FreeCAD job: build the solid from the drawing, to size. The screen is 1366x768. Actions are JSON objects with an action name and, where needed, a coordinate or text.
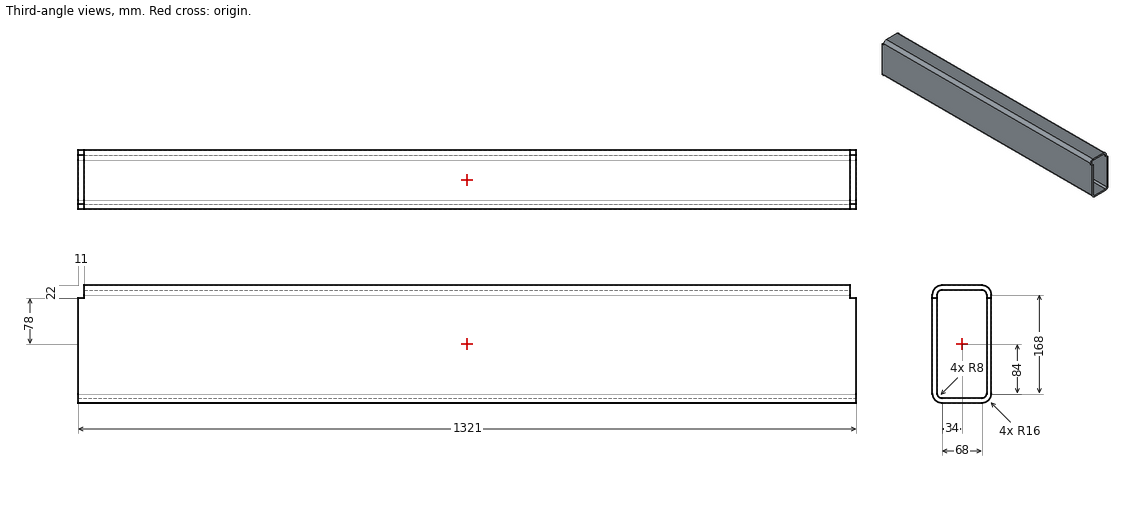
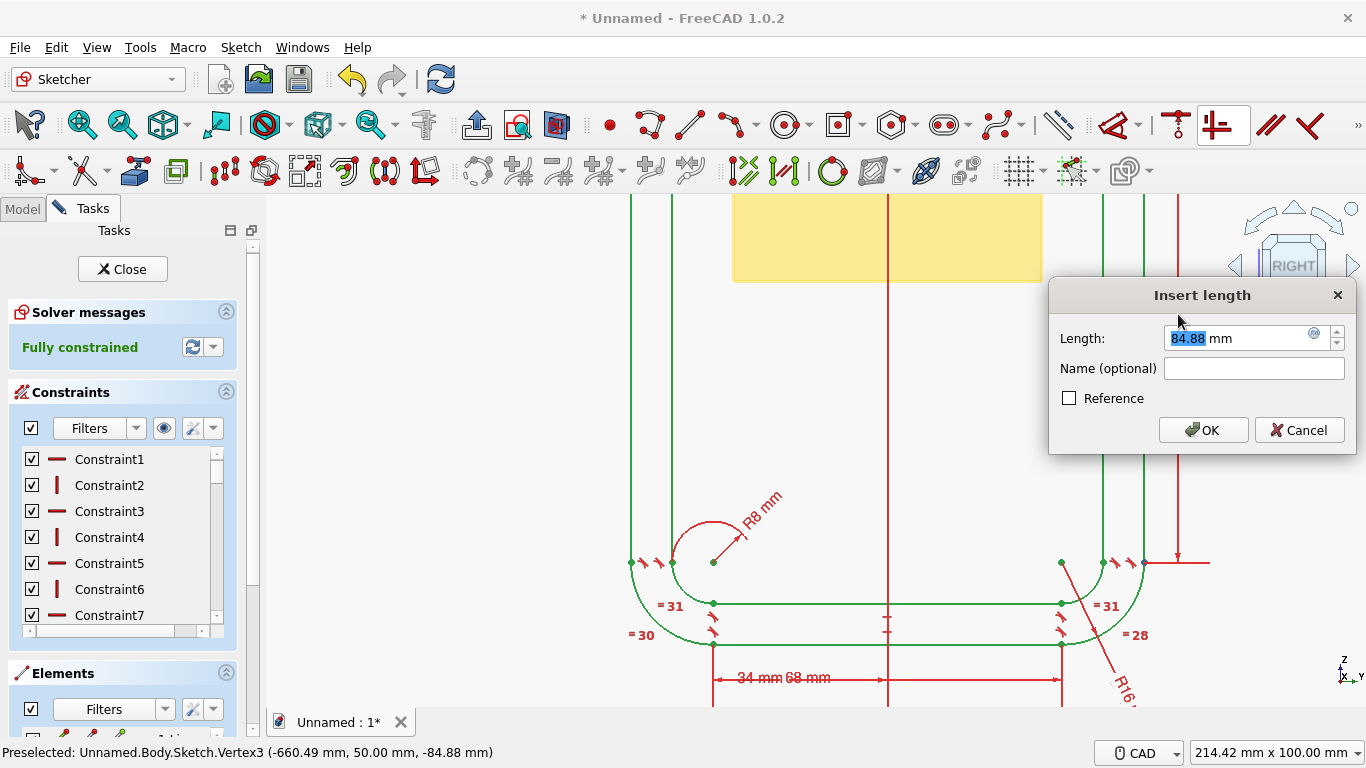
{"action": "type", "text": "84"}
{"action": "key", "text": "Return"}
{"action": "key", "text": "Escape"}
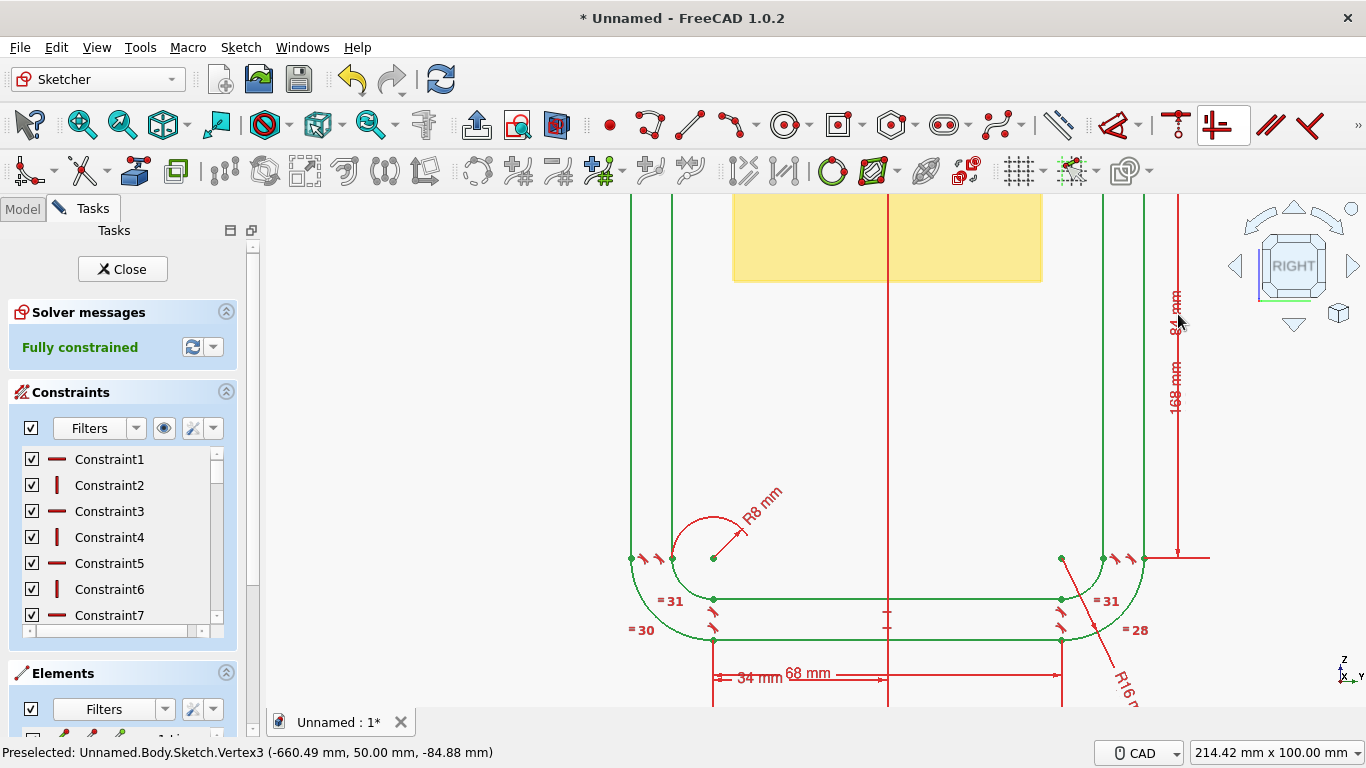
{"action": "left_click", "coordinate": [123, 269]}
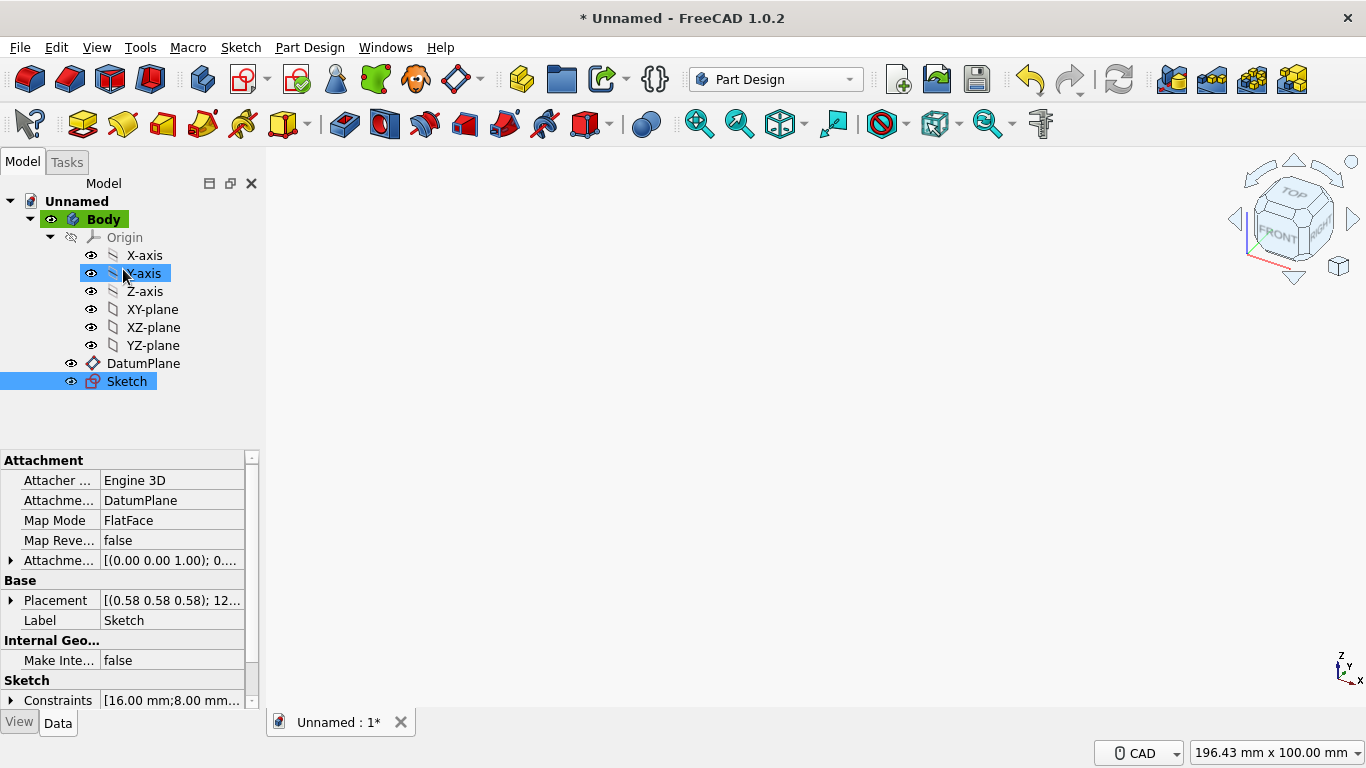
{"action": "left_click", "coordinate": [84, 124]}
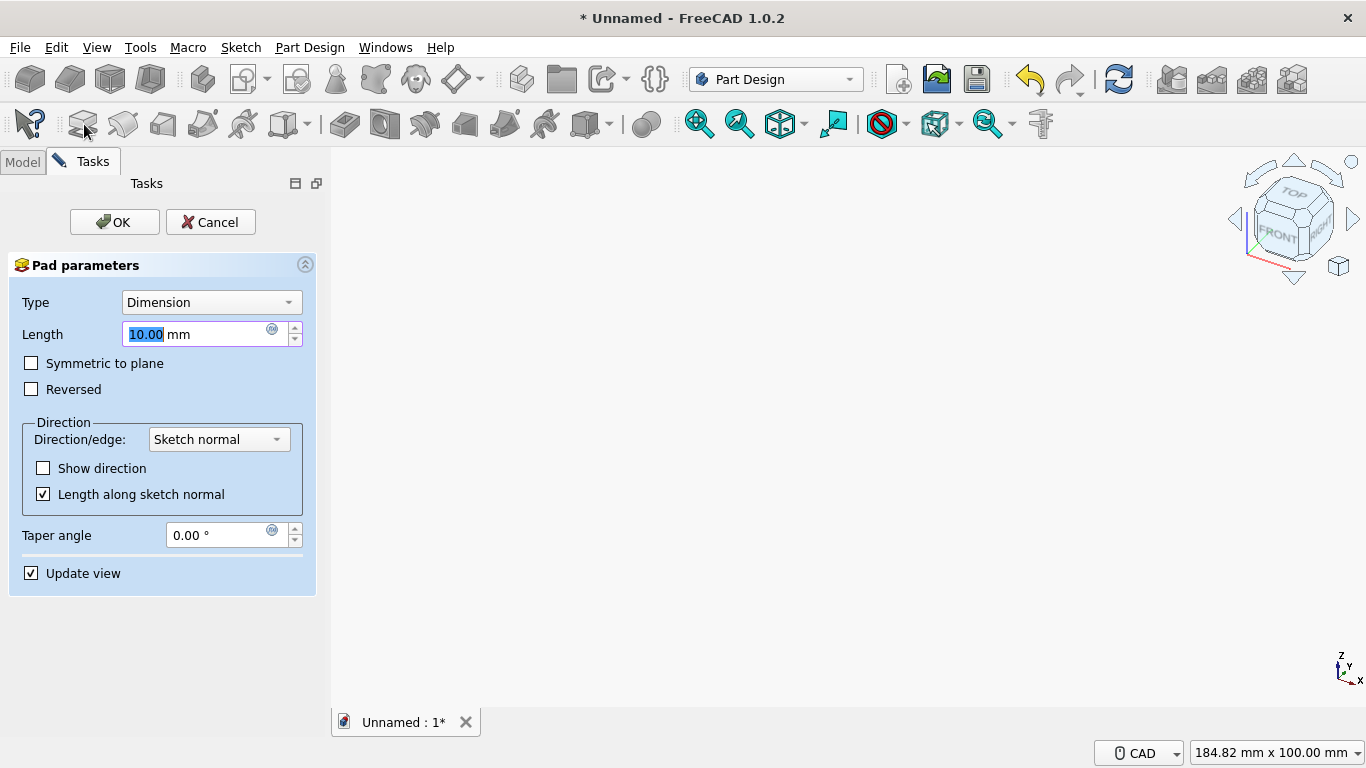
{"action": "type", "text": "1321"}
{"action": "key", "text": "Tab"}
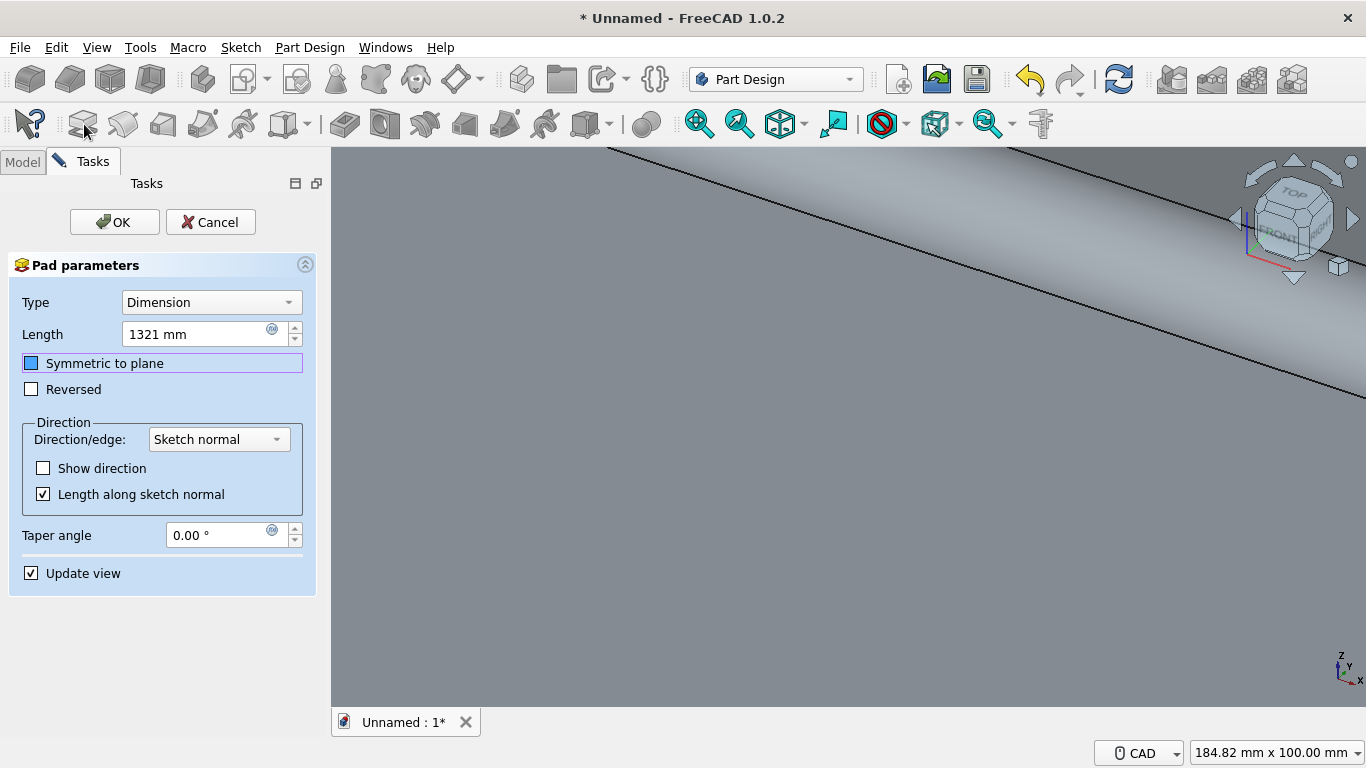
{"action": "left_click", "coordinate": [115, 222]}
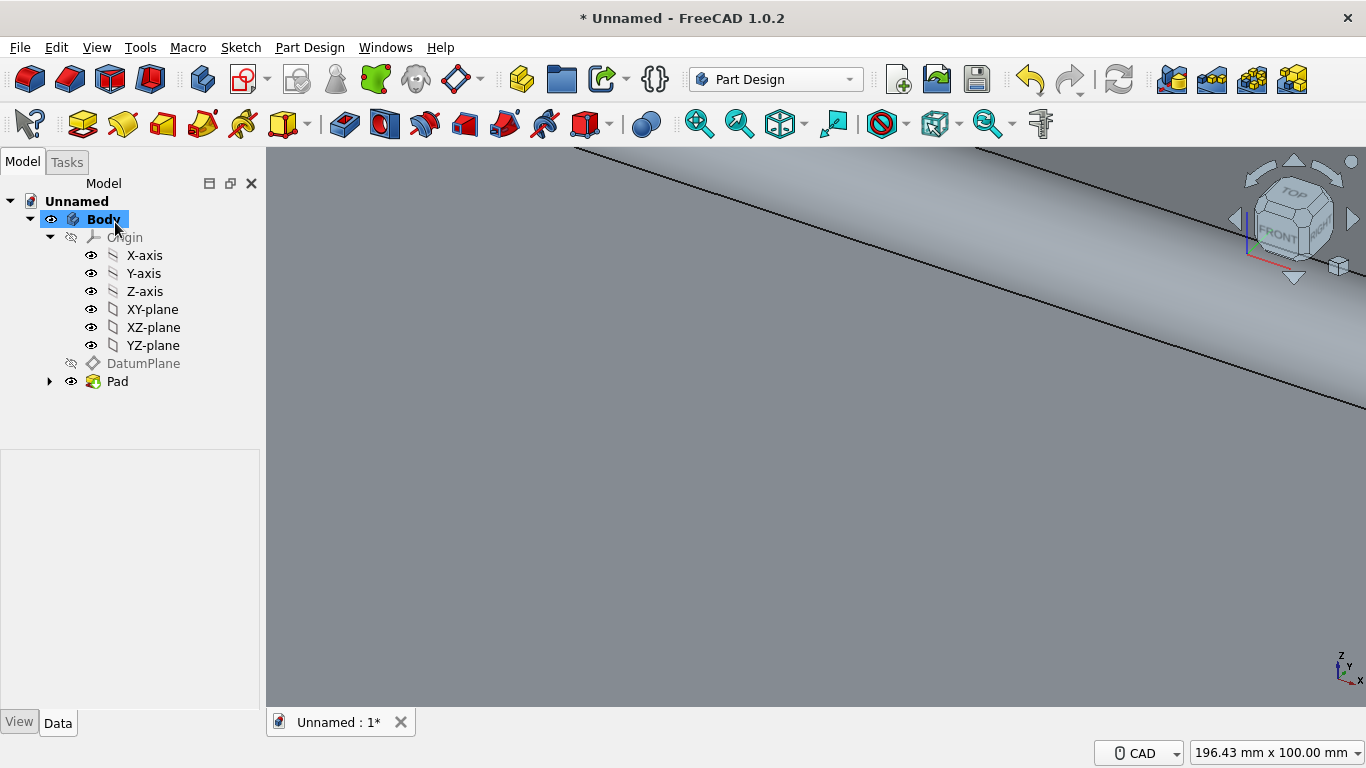
{"action": "key", "text": "v f"}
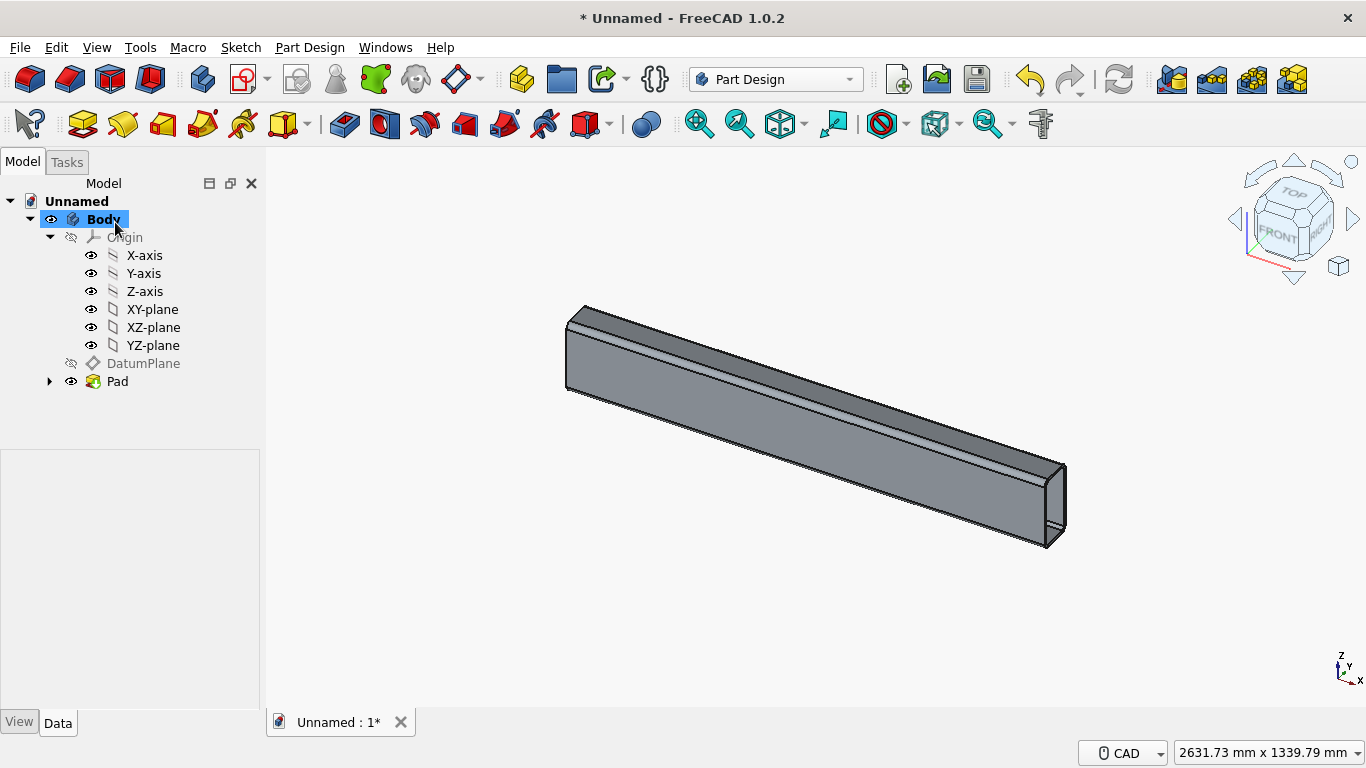
{"action": "left_click", "coordinate": [806, 436]}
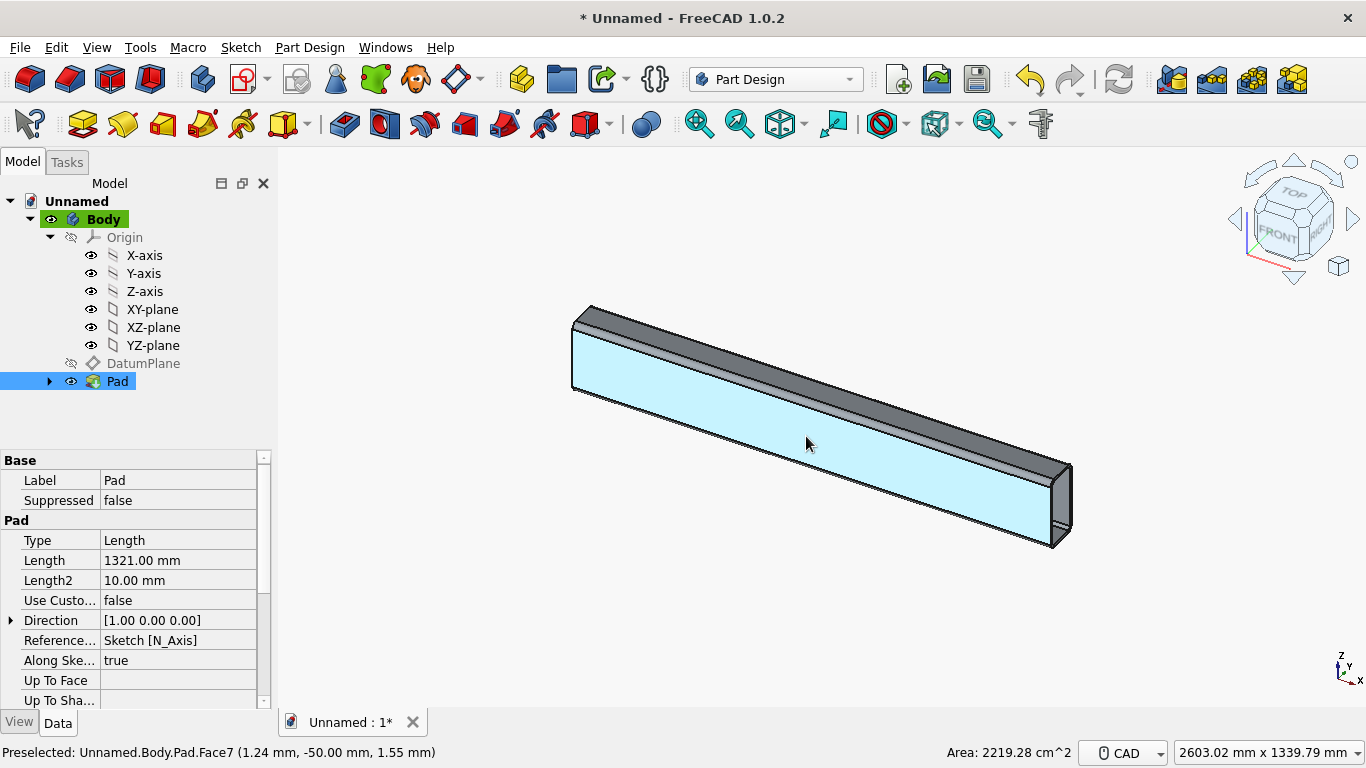
{"action": "left_click", "coordinate": [244, 80]}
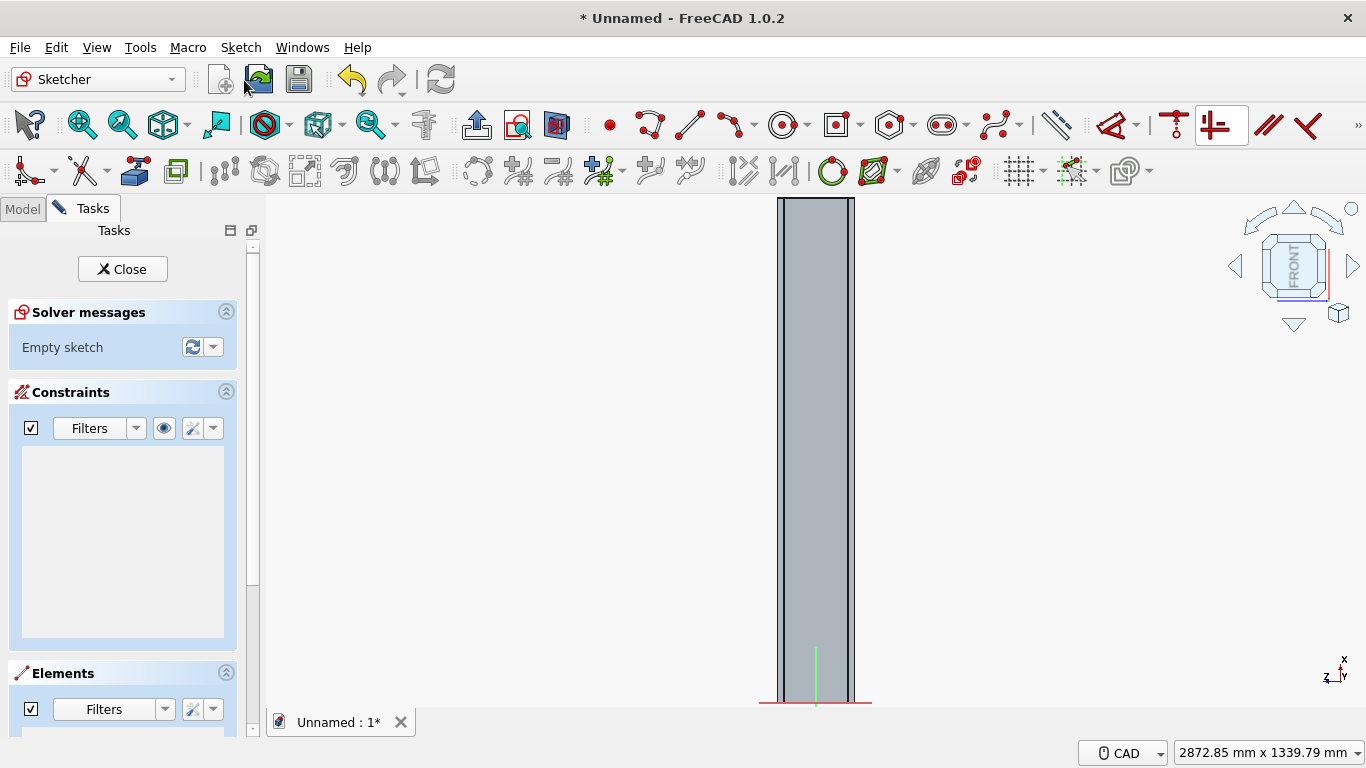
{"action": "scroll", "coordinate": [748, 450], "scroll_direction": "down", "scroll_amount": 5}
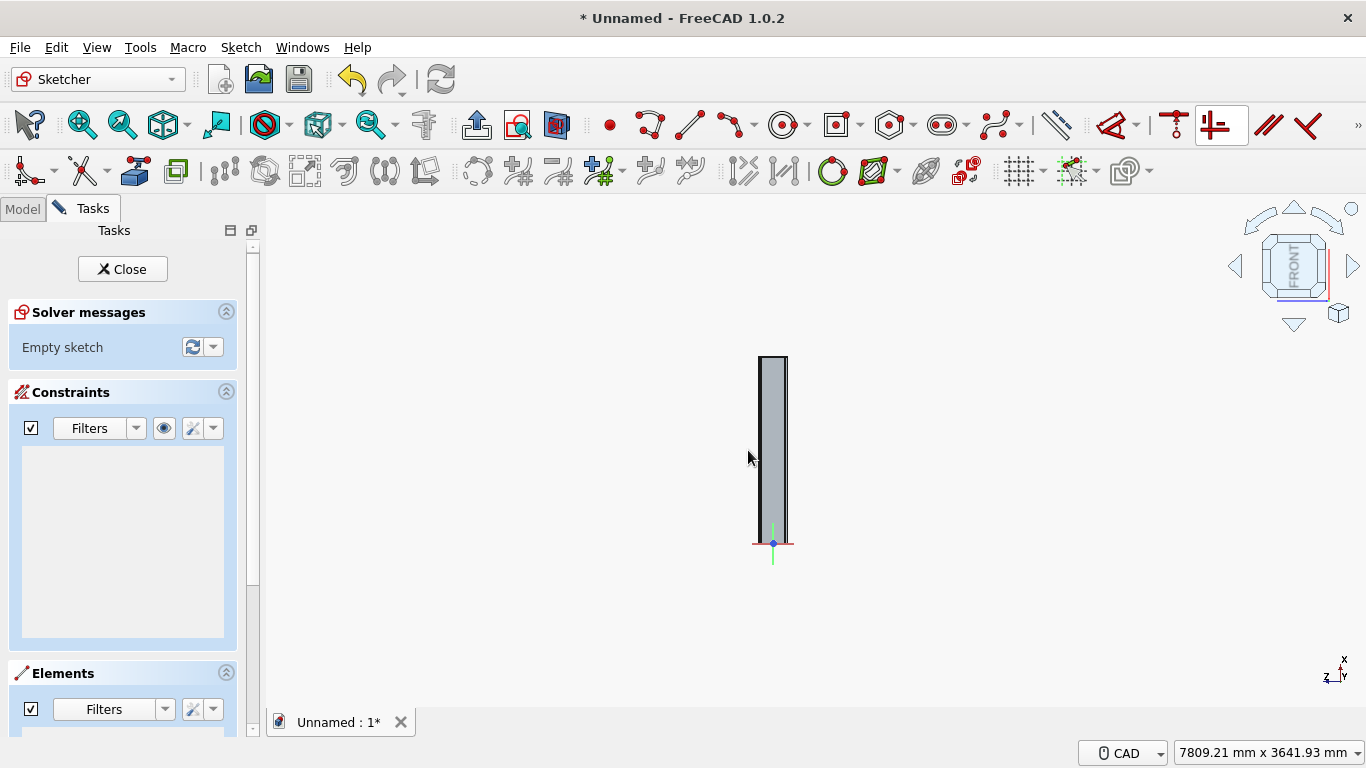
{"action": "scroll", "coordinate": [761, 548], "scroll_direction": "up", "scroll_amount": 15}